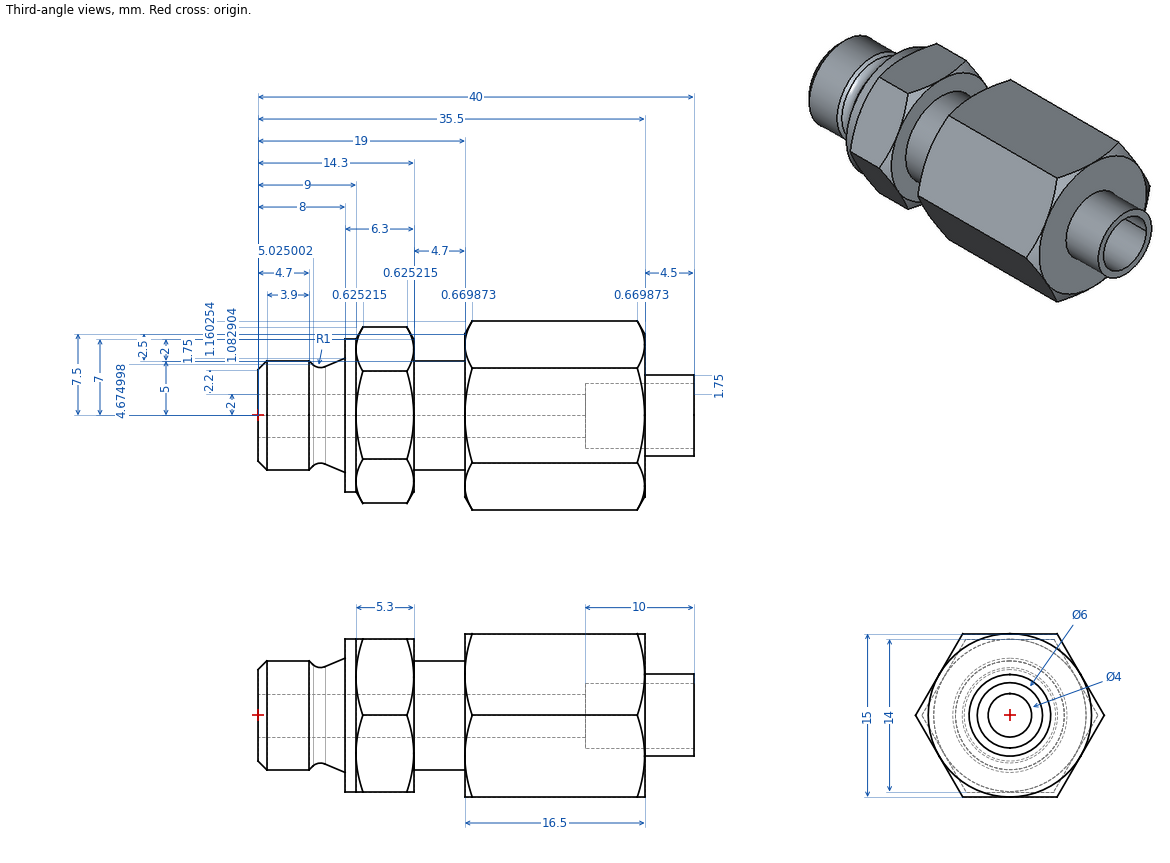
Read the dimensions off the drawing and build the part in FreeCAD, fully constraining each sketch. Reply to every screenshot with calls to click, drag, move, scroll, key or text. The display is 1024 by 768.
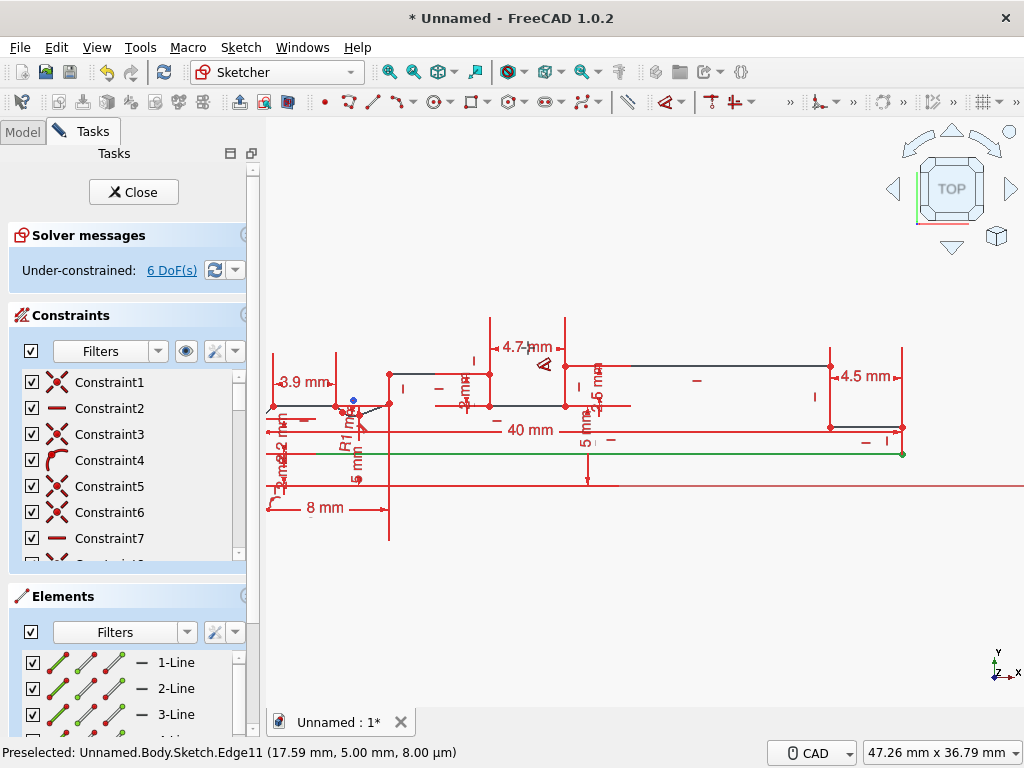
click(460, 374)
click(439, 340)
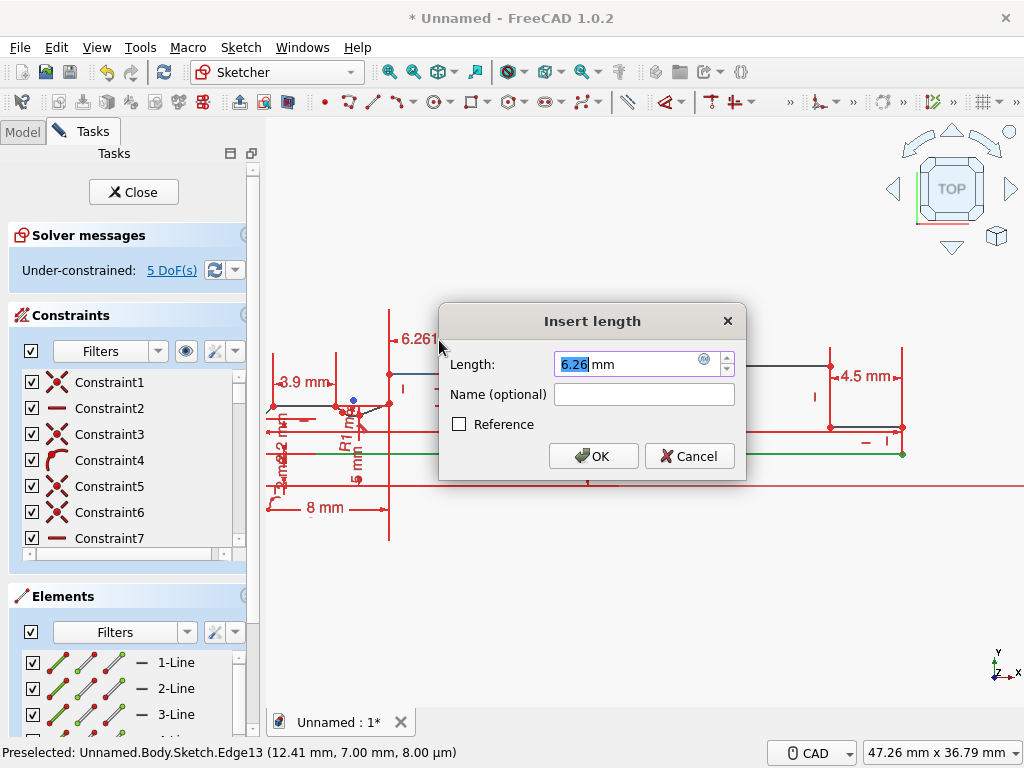
text(6.3)
key(Return)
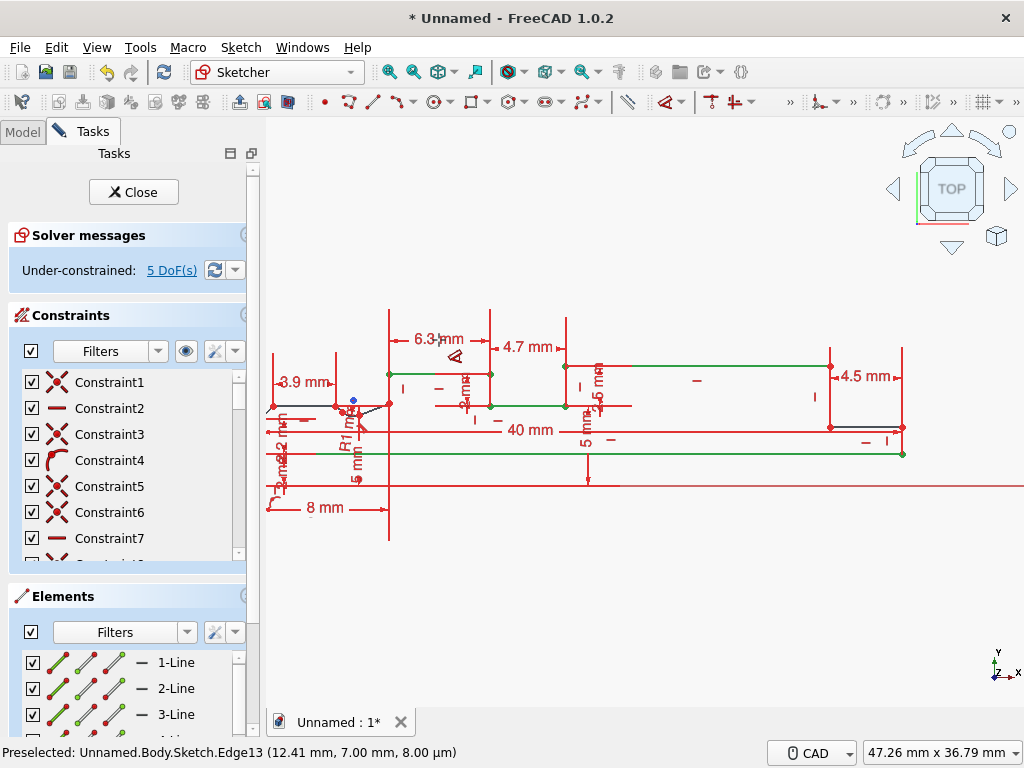
scroll(566, 383, down, 2)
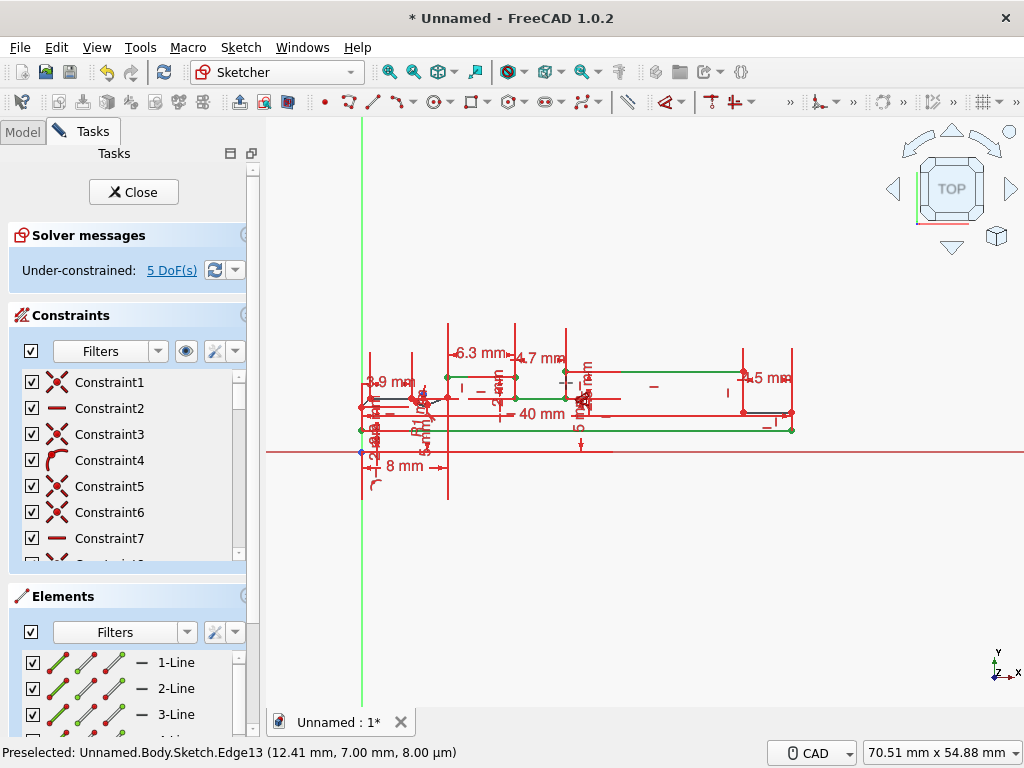
scroll(792, 424, up, 4)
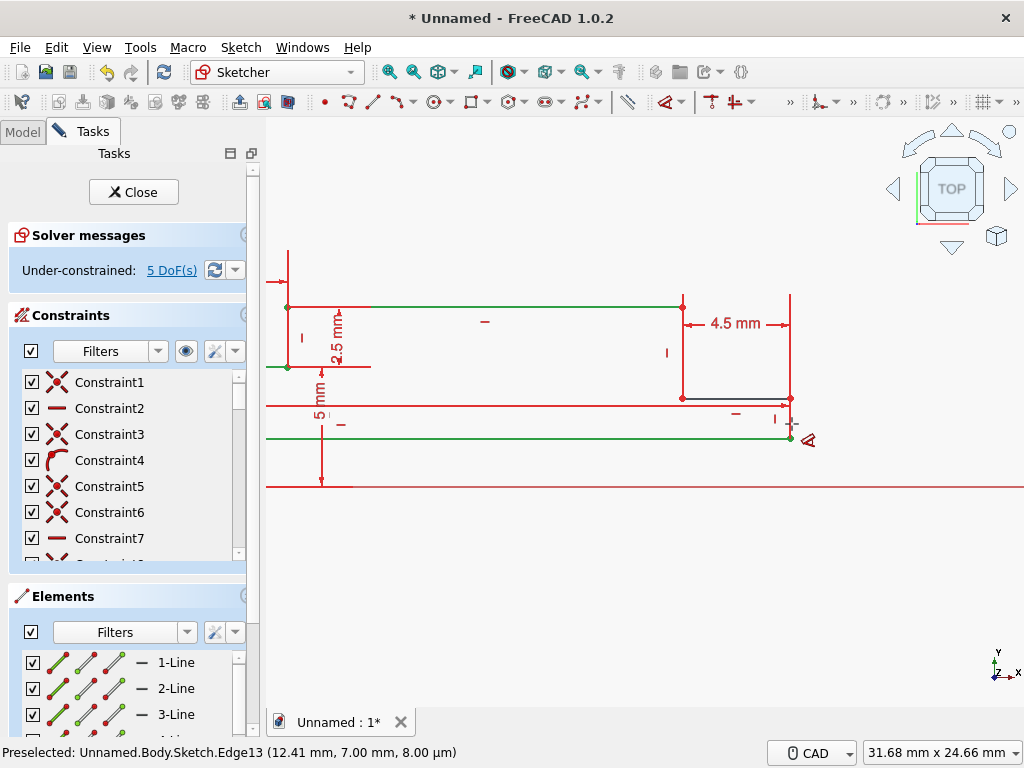
click(790, 423)
click(824, 419)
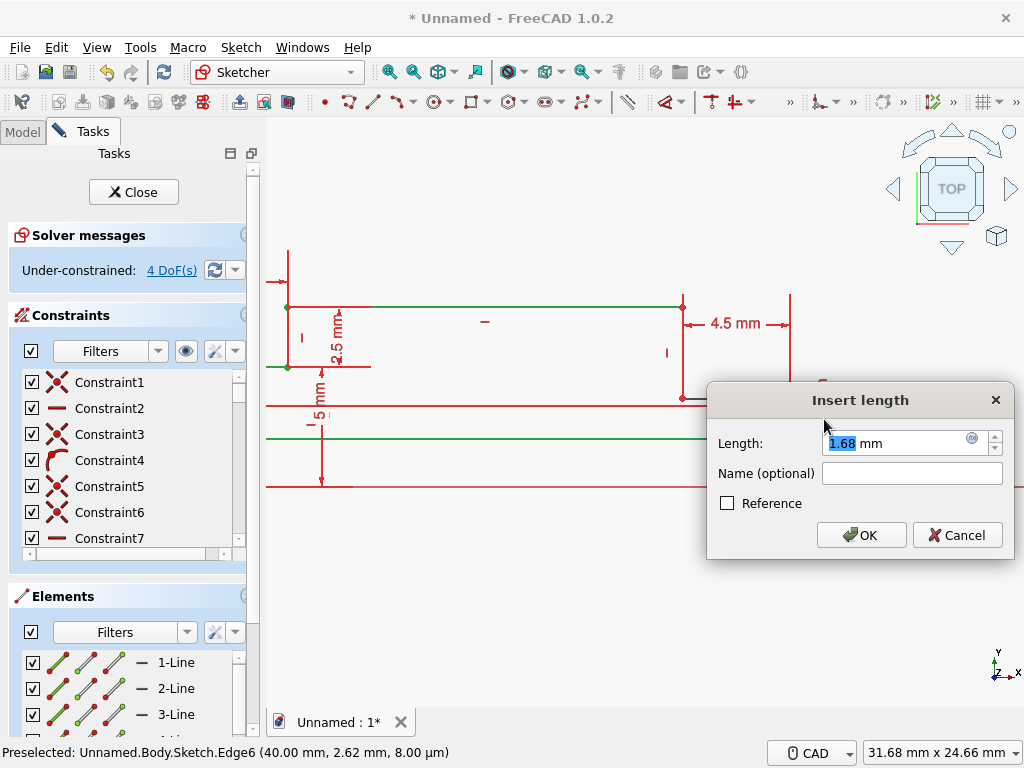
text(1.75)
key(Return)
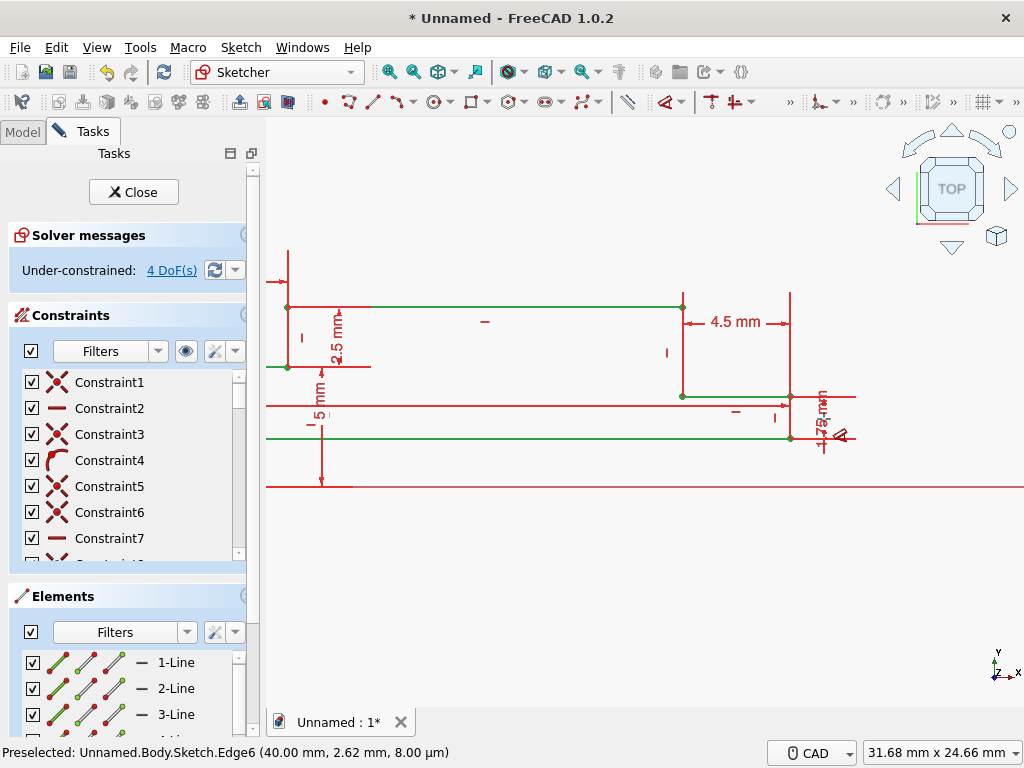
scroll(792, 424, down, 4)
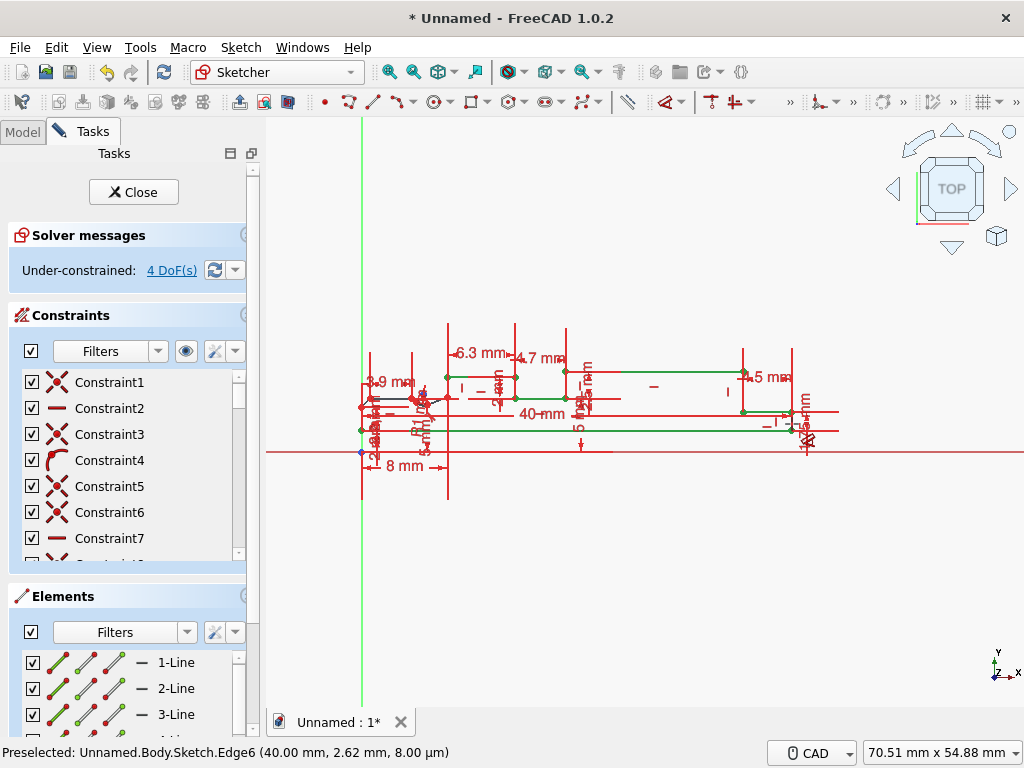
scroll(448, 383, up, 5)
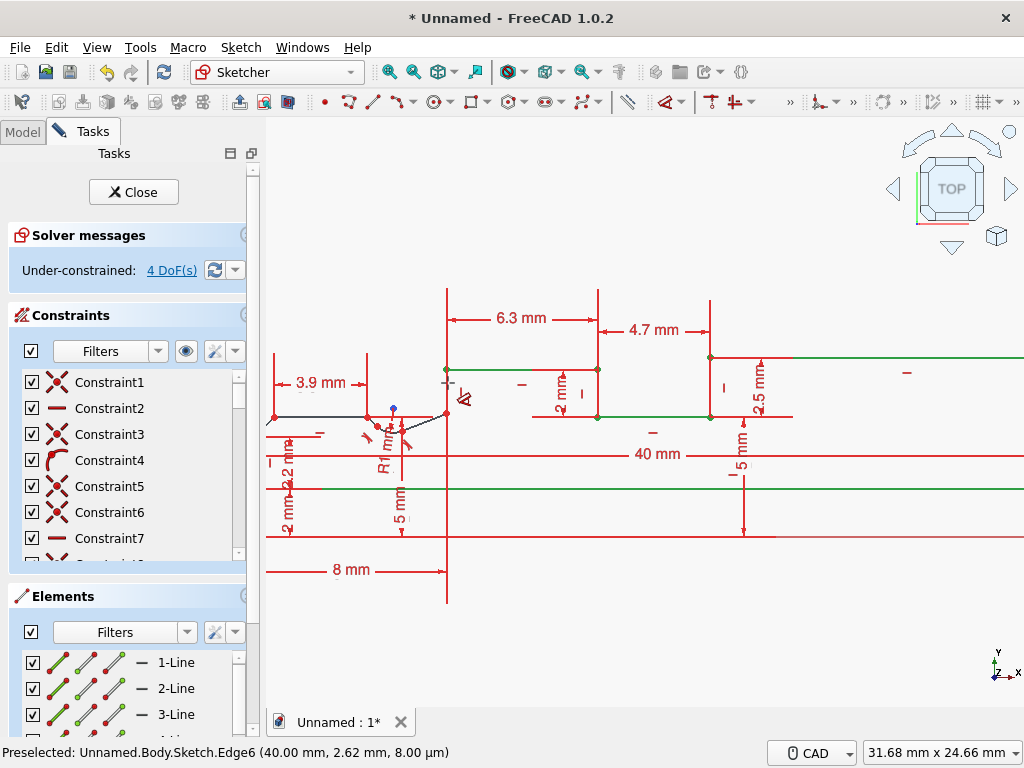
click(447, 383)
click(413, 393)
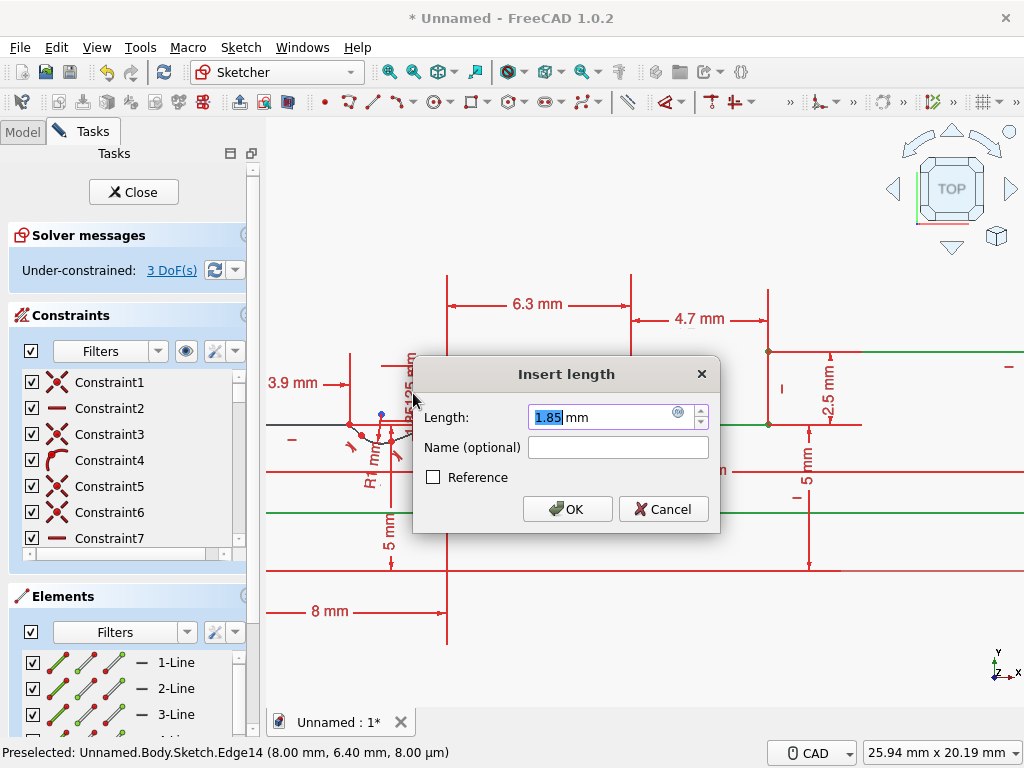
text(1.75)
key(Return)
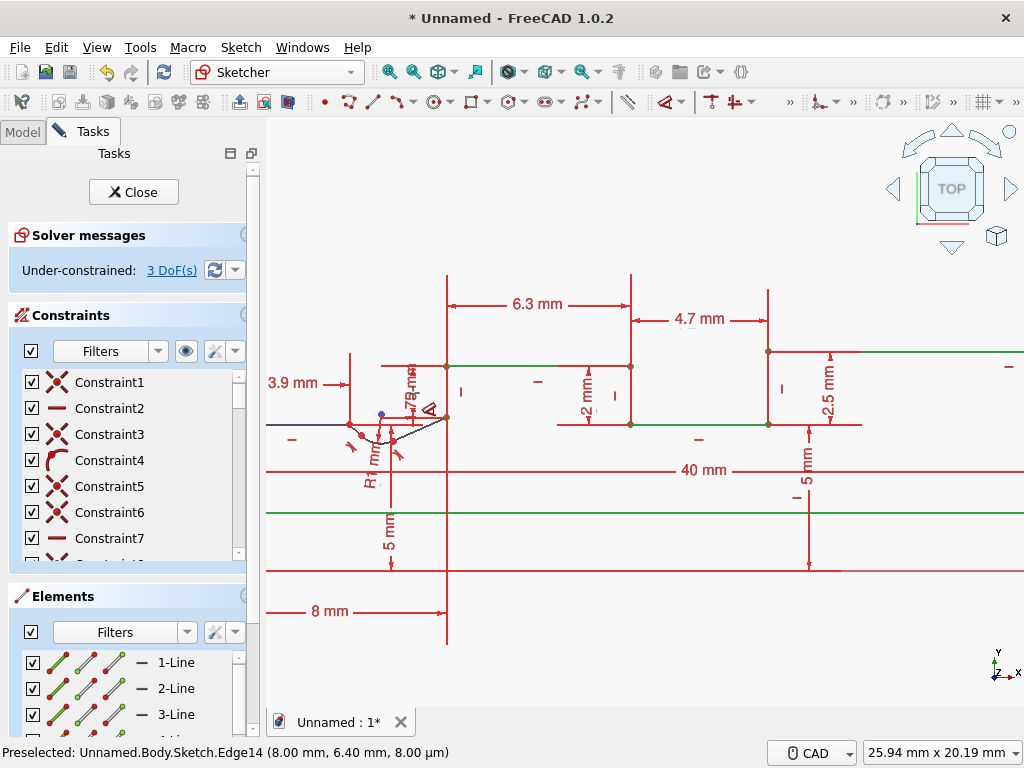
click(350, 425)
click(322, 653)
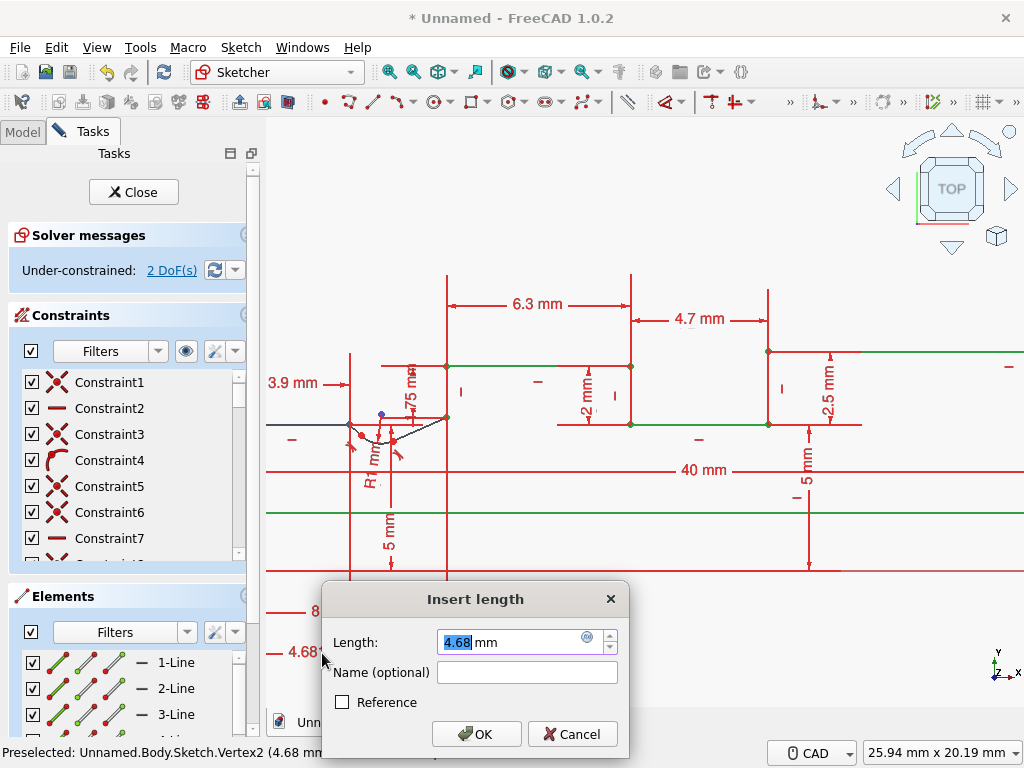
text(4.7)
key(Return)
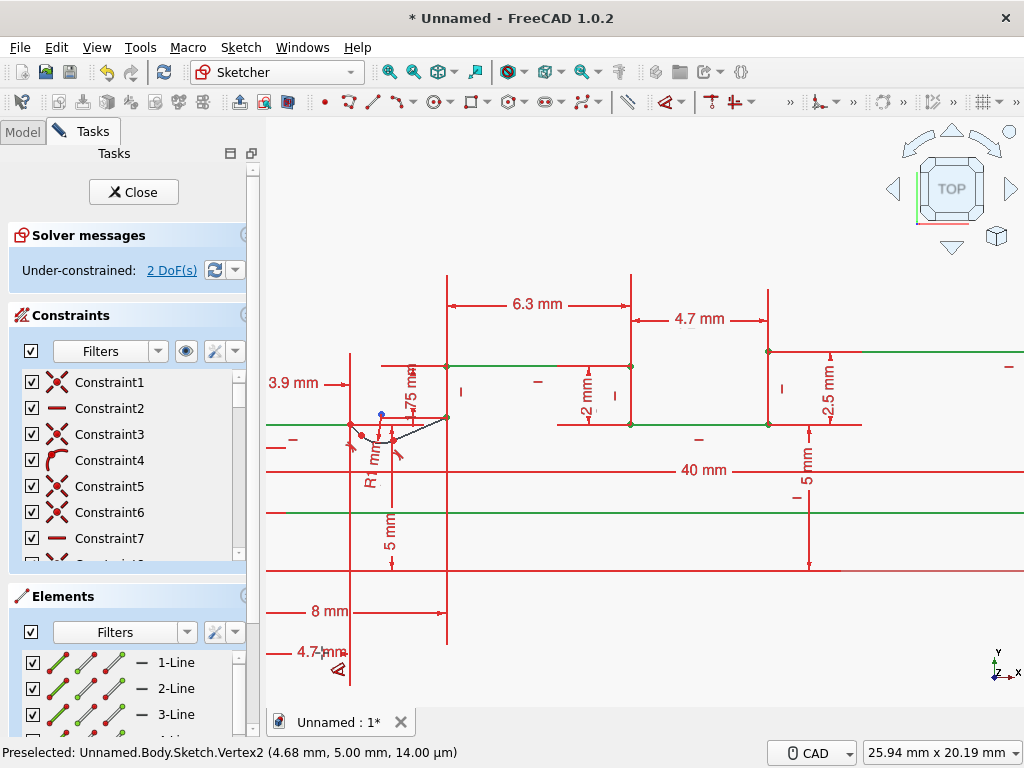
click(361, 435)
click(328, 353)